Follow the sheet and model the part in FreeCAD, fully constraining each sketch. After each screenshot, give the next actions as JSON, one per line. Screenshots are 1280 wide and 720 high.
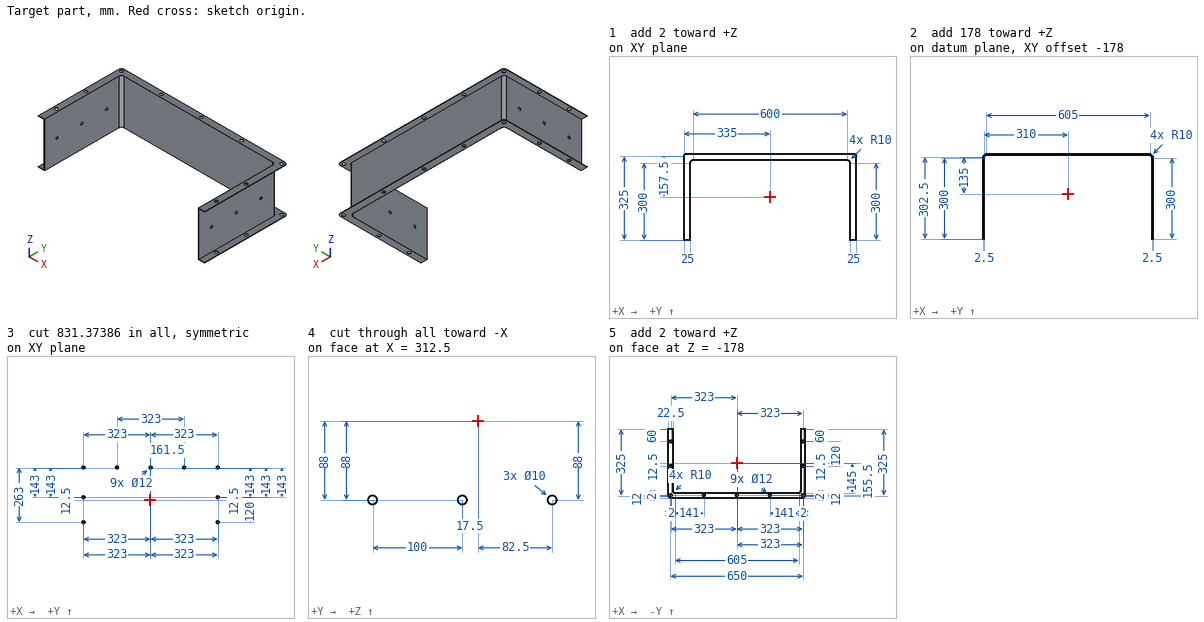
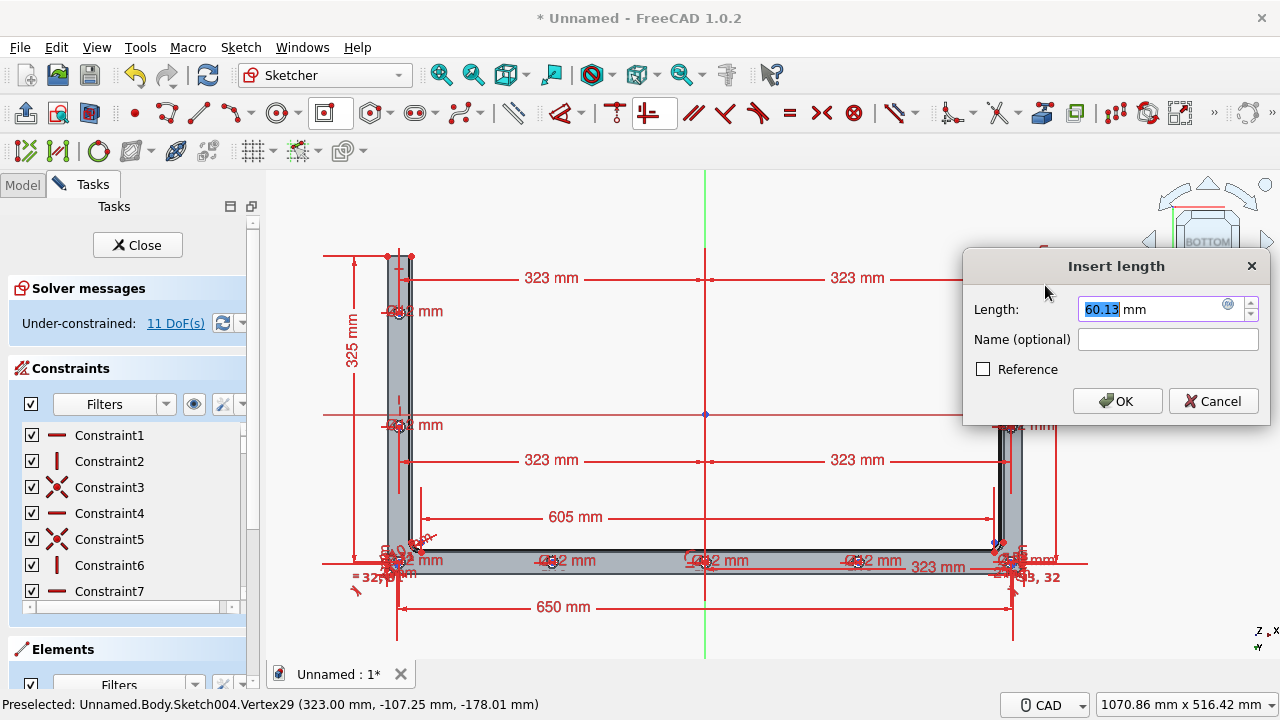
{"action": "type", "text": "60"}
{"action": "key", "text": "Return"}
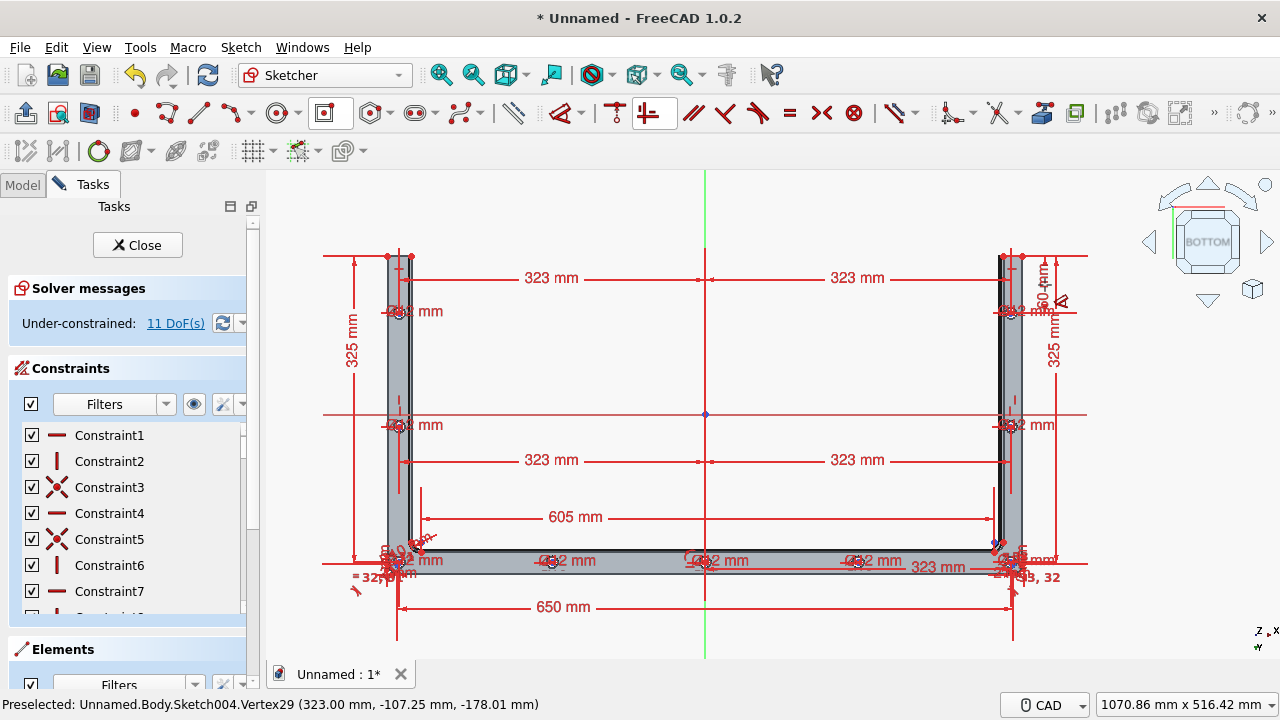
{"action": "left_click", "coordinate": [412, 256]}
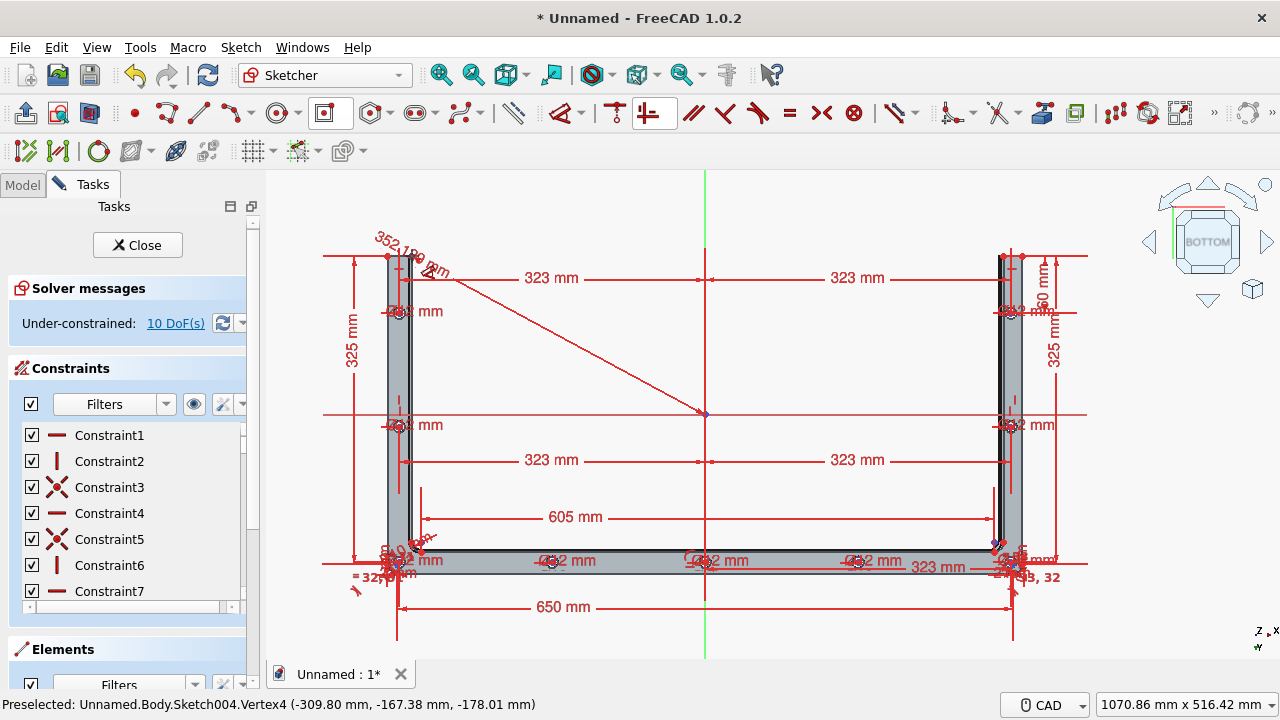
{"action": "left_click", "coordinate": [399, 313]}
{"action": "left_click", "coordinate": [365, 285]}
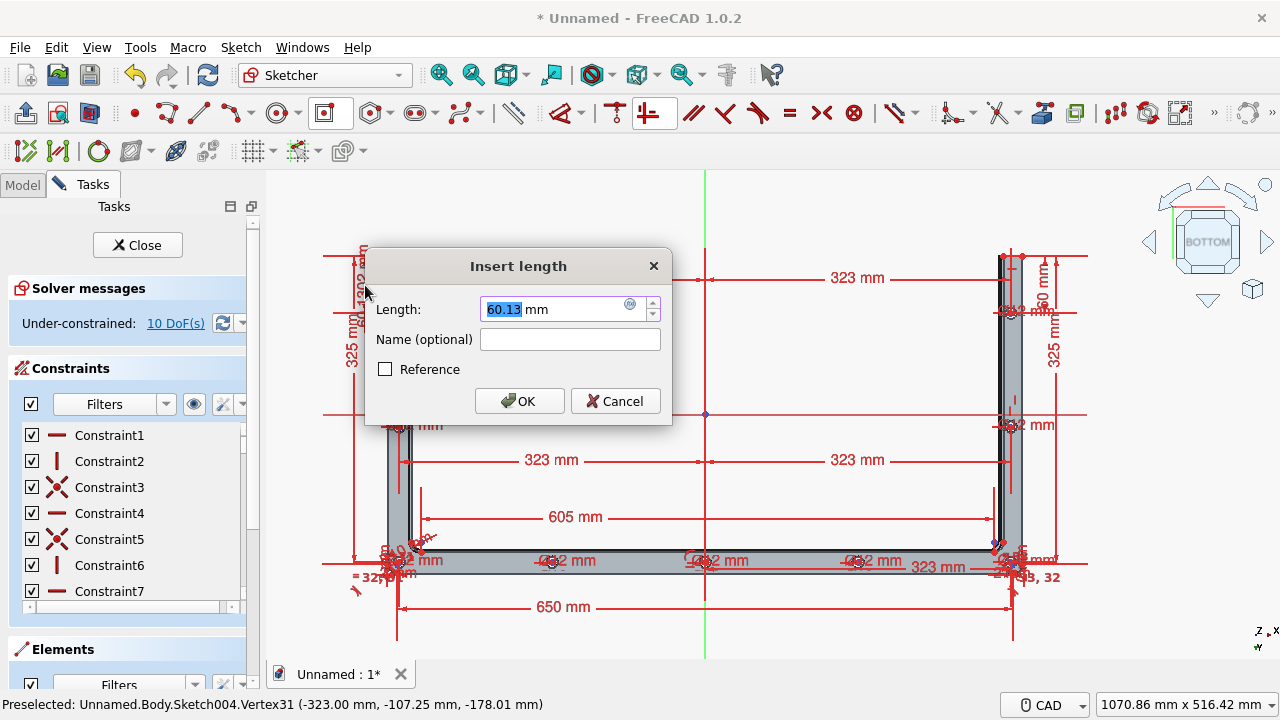
{"action": "type", "text": "60"}
{"action": "key", "text": "Return"}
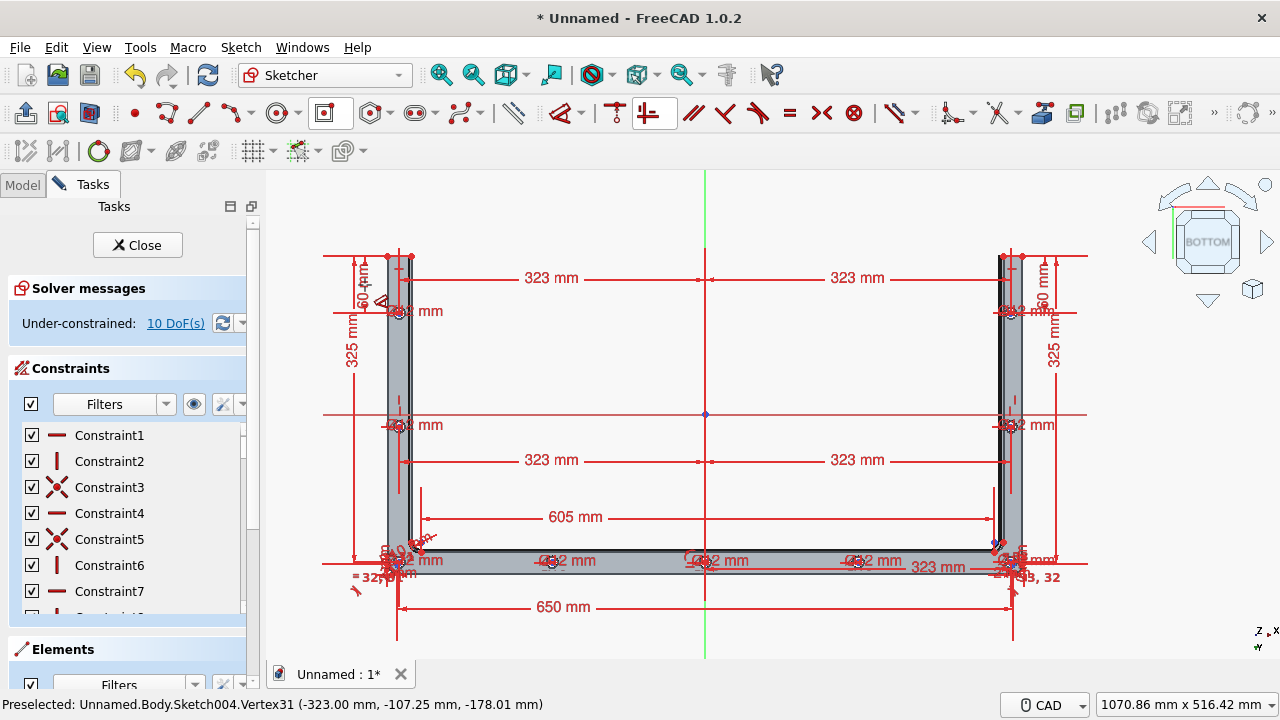
{"action": "scroll", "coordinate": [1013, 574], "scroll_direction": "up", "scroll_amount": 7}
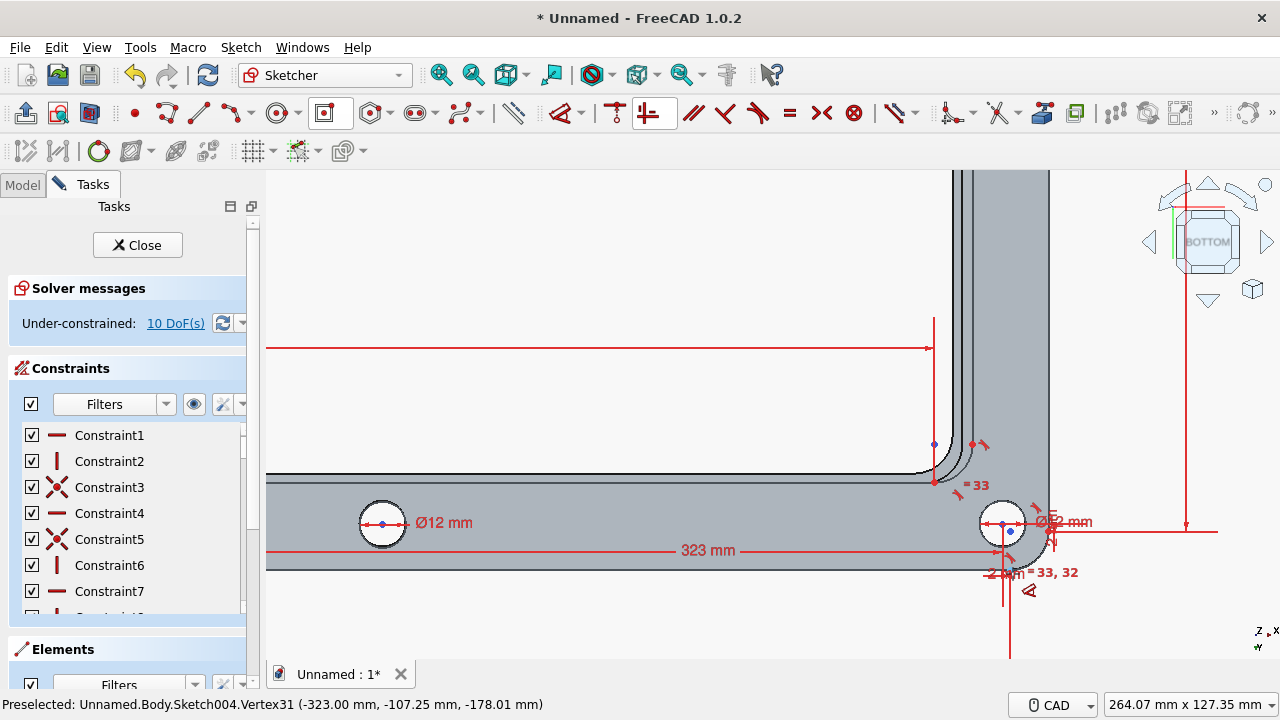
{"action": "left_click", "coordinate": [1010, 570]}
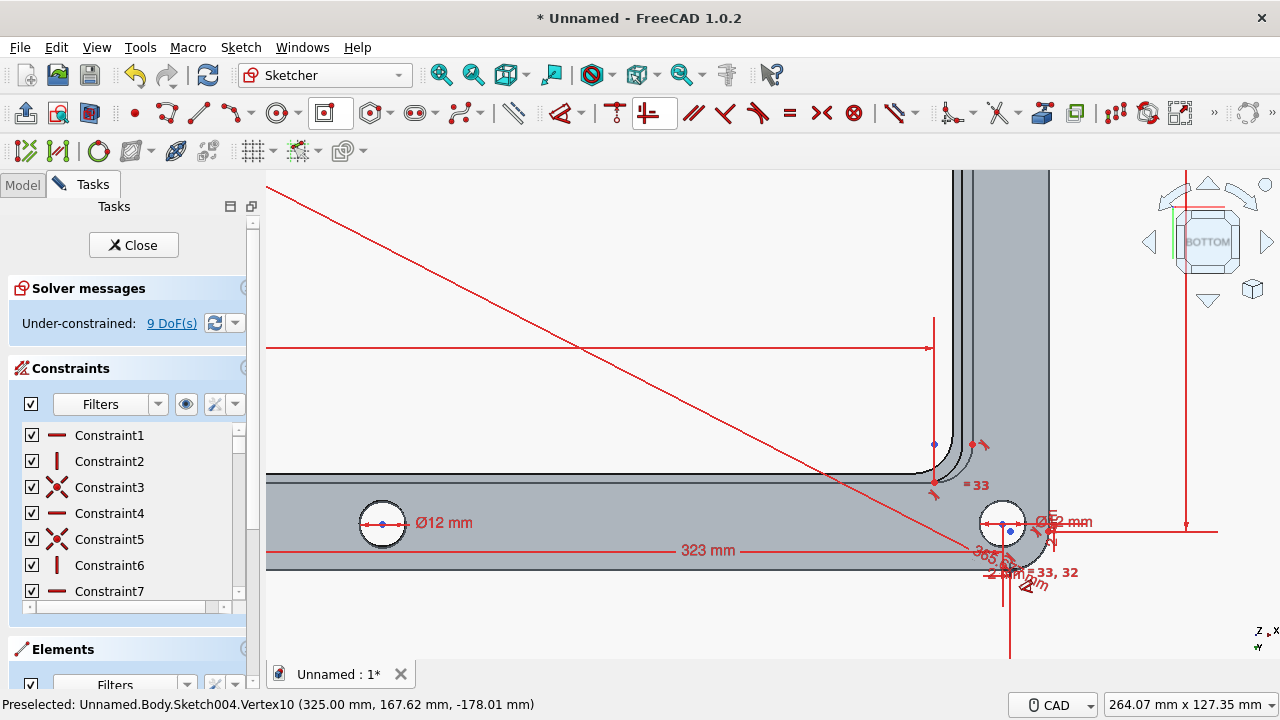
{"action": "left_click", "coordinate": [383, 525]}
{"action": "left_click", "coordinate": [349, 548]}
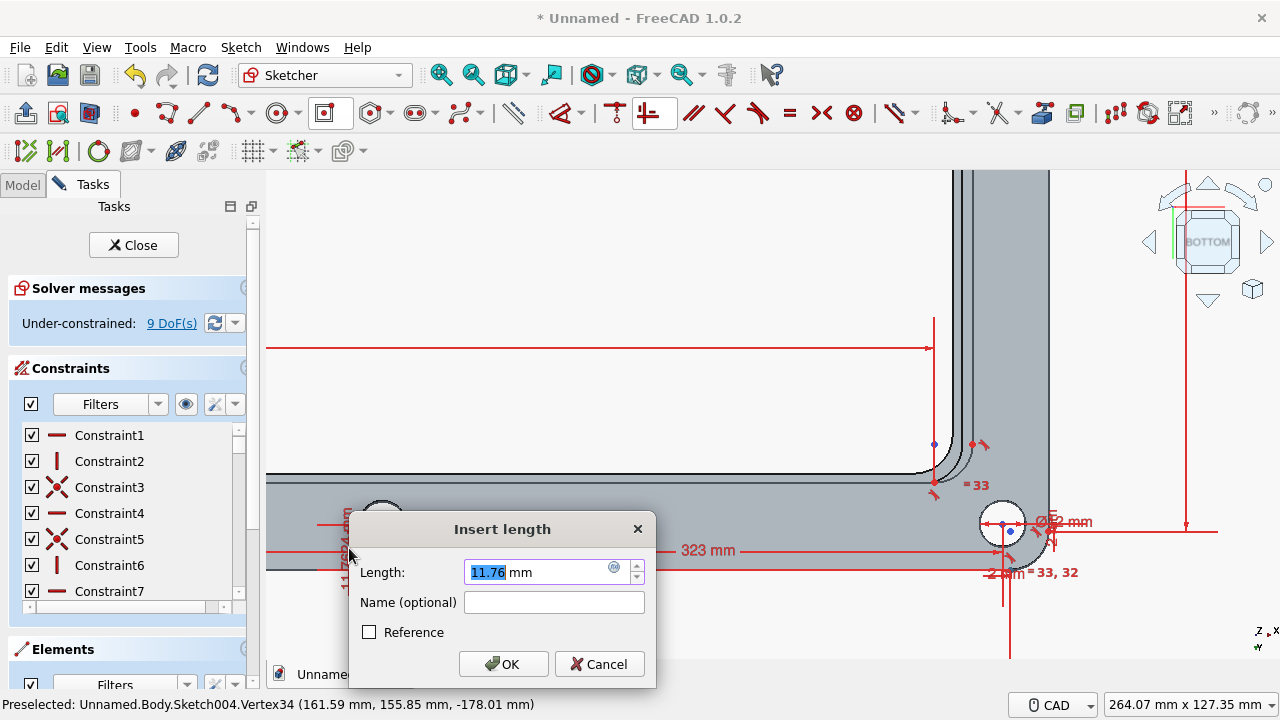
{"action": "type", "text": "12"}
{"action": "key", "text": "Return"}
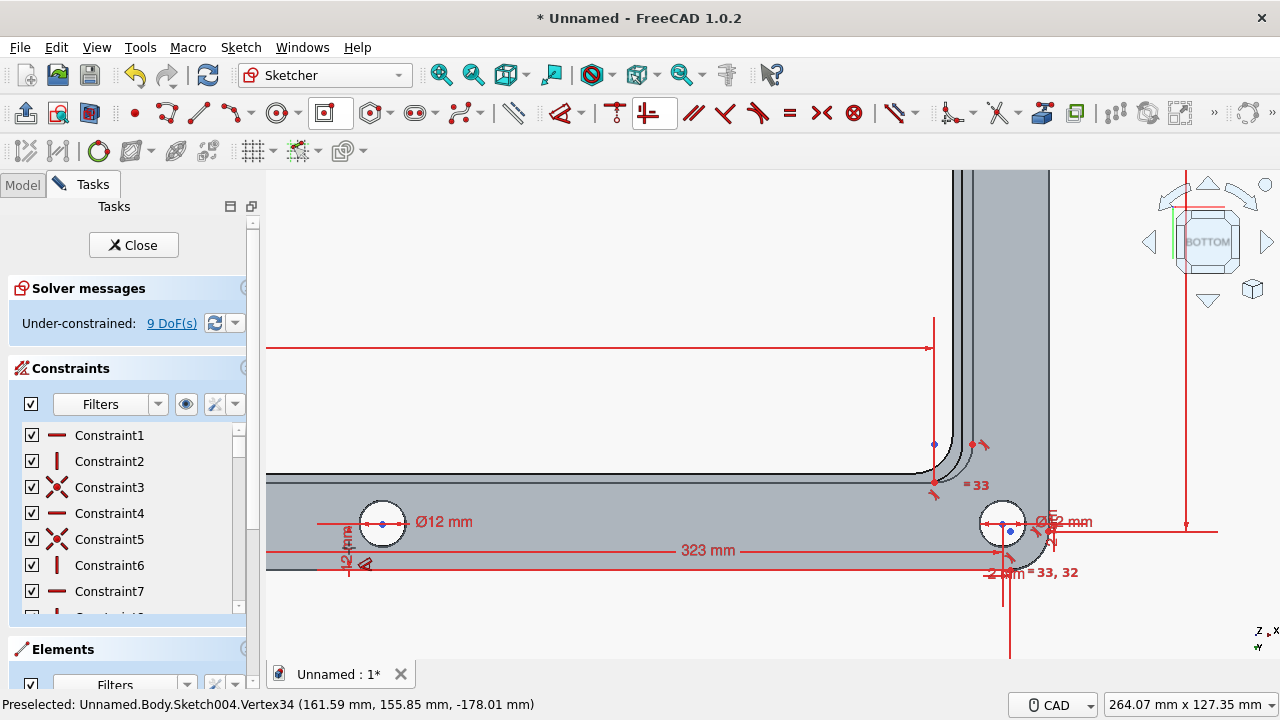
{"action": "scroll", "coordinate": [1013, 574], "scroll_direction": "down", "scroll_amount": 7}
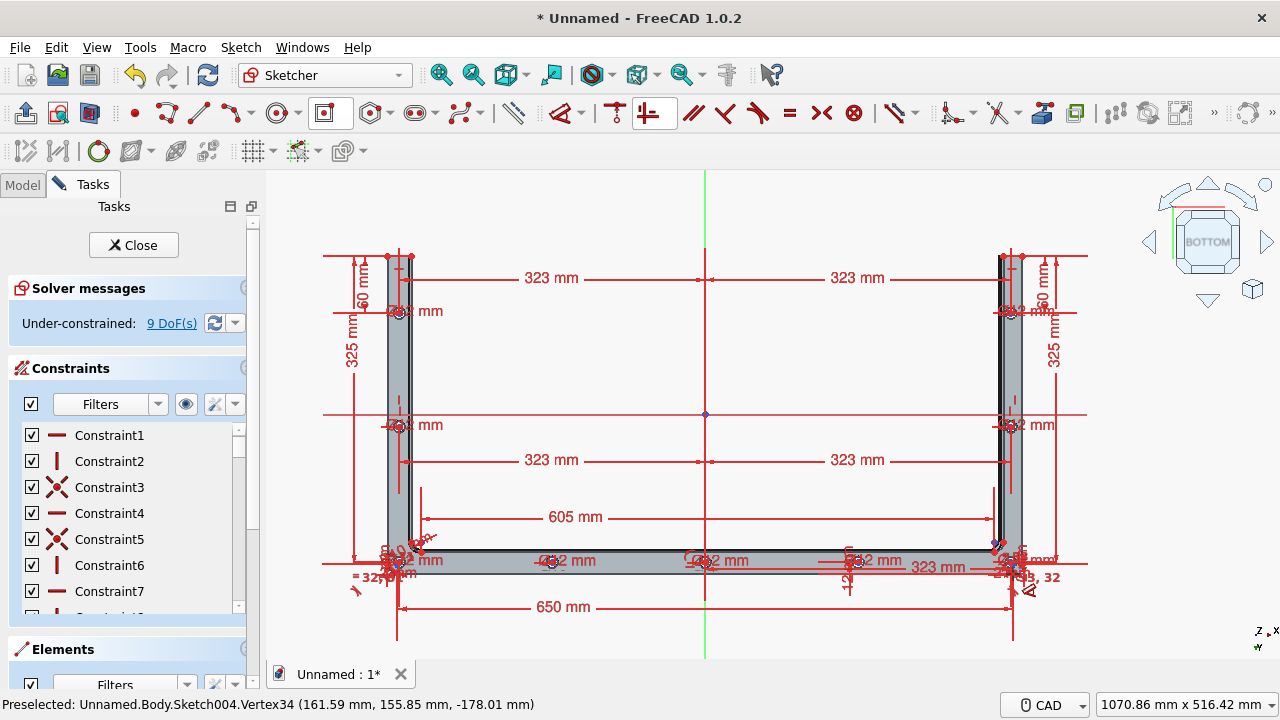
{"action": "scroll", "coordinate": [397, 574], "scroll_direction": "up", "scroll_amount": 7}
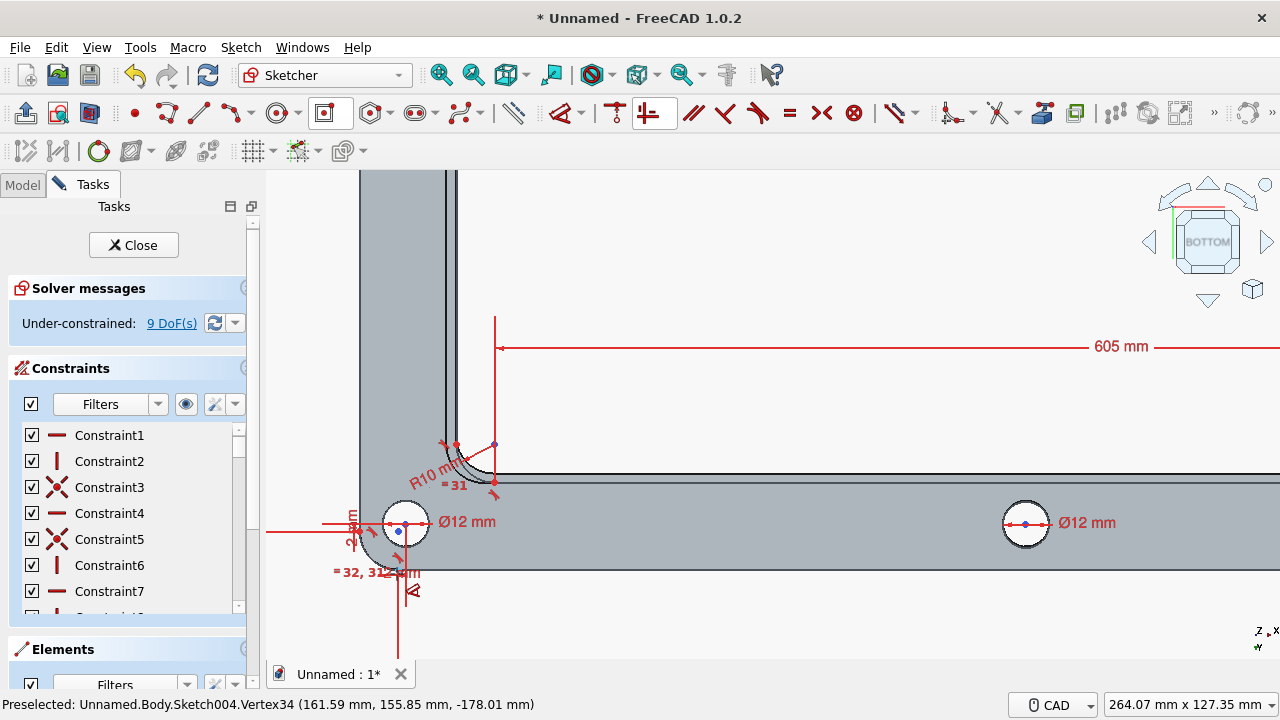
{"action": "left_click", "coordinate": [398, 570]}